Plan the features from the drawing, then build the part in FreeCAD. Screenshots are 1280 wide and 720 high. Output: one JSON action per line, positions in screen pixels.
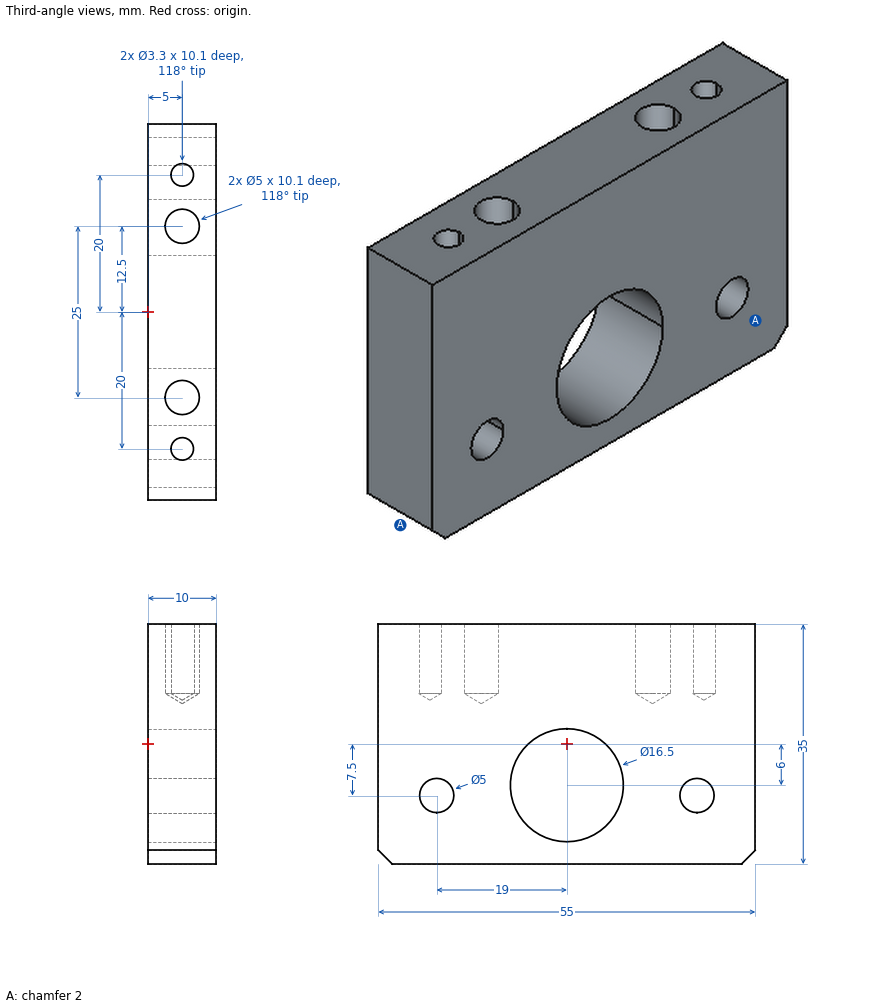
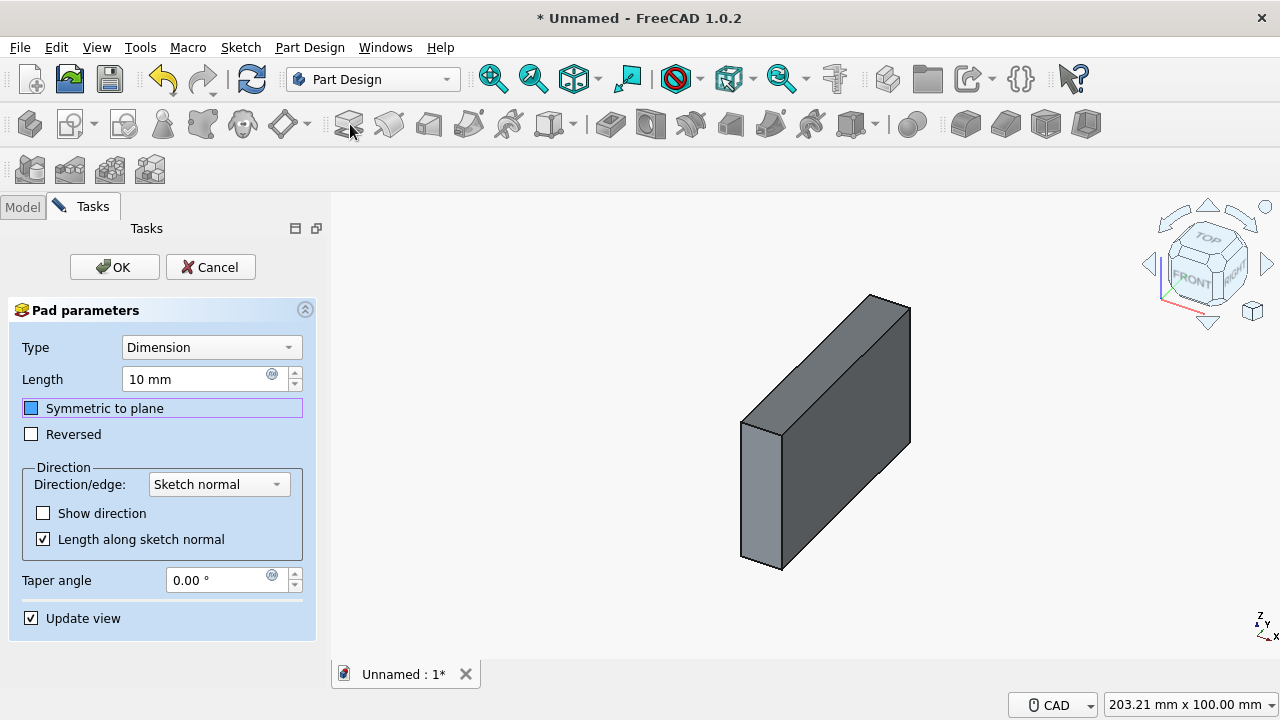
{"action": "left_click", "coordinate": [115, 267]}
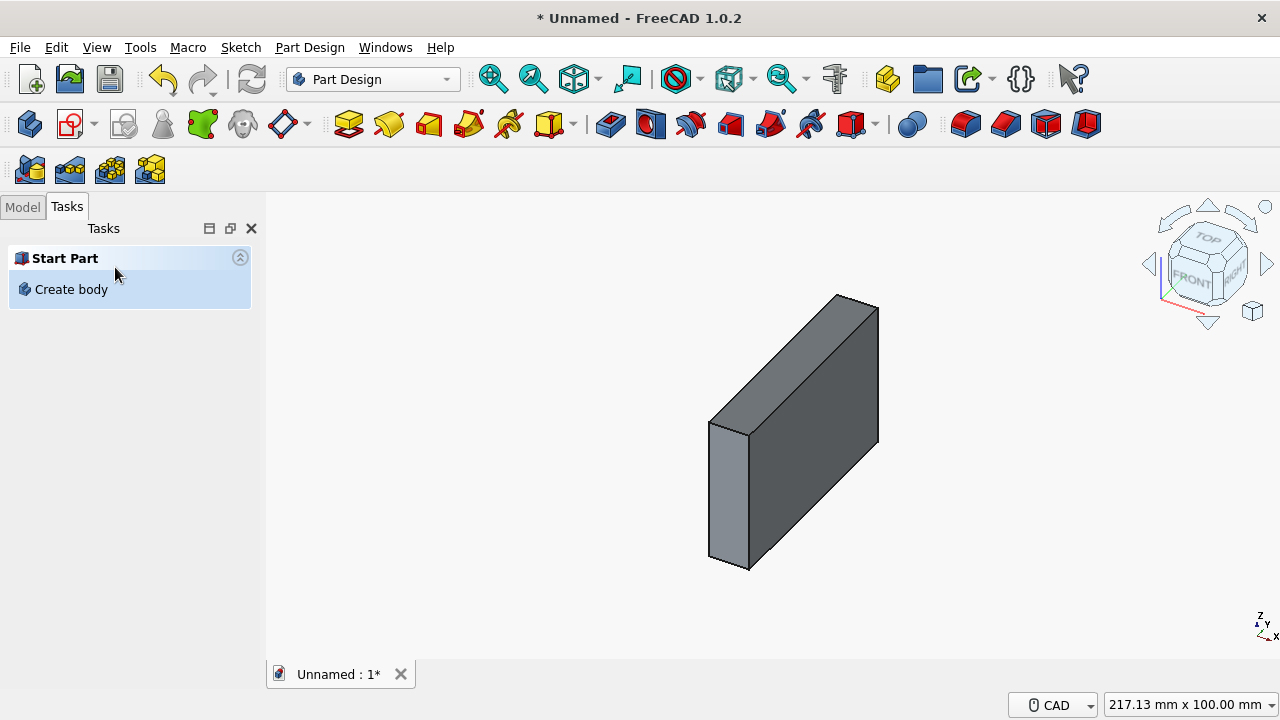
{"action": "left_click", "coordinate": [70, 124]}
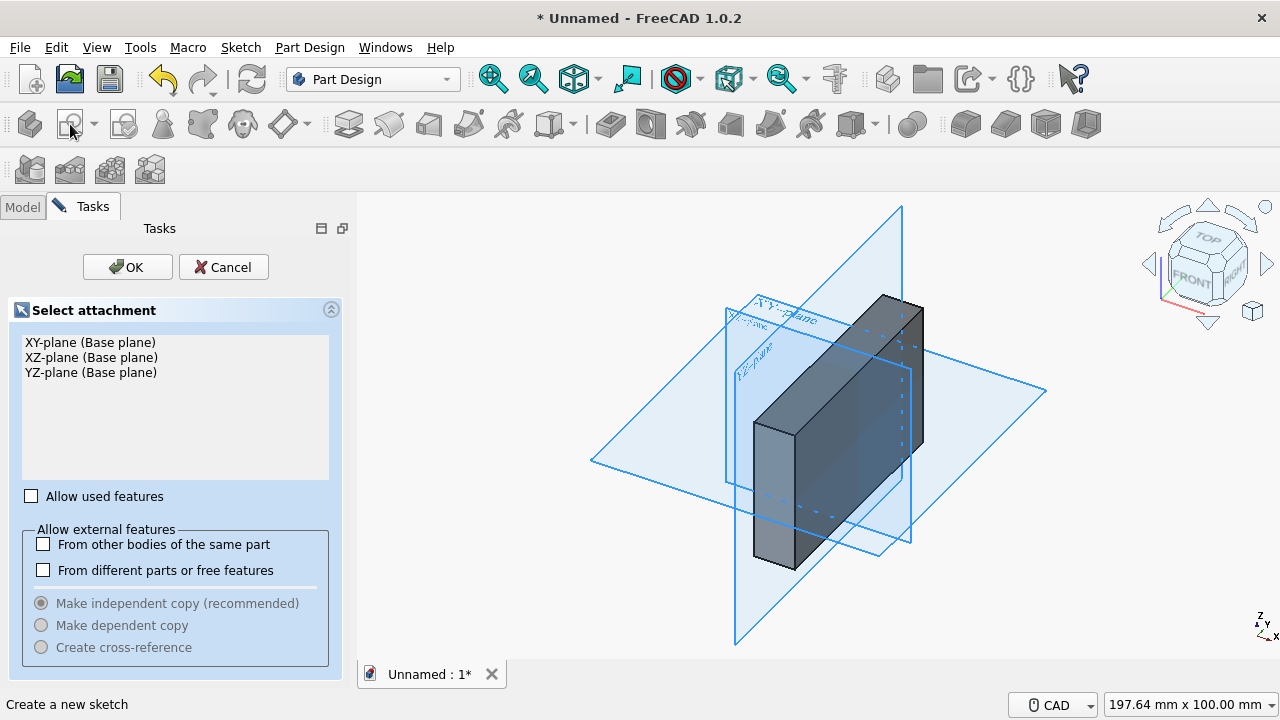
{"action": "left_click", "coordinate": [82, 372]}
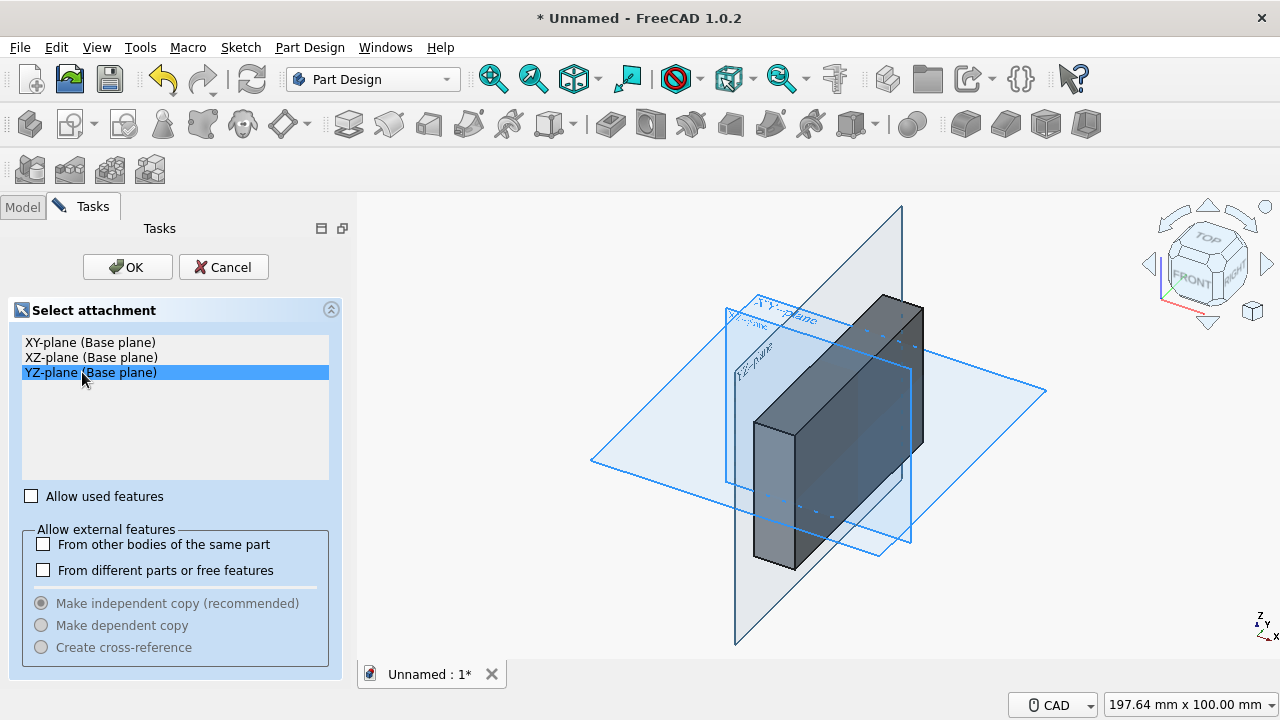
{"action": "left_click", "coordinate": [128, 267]}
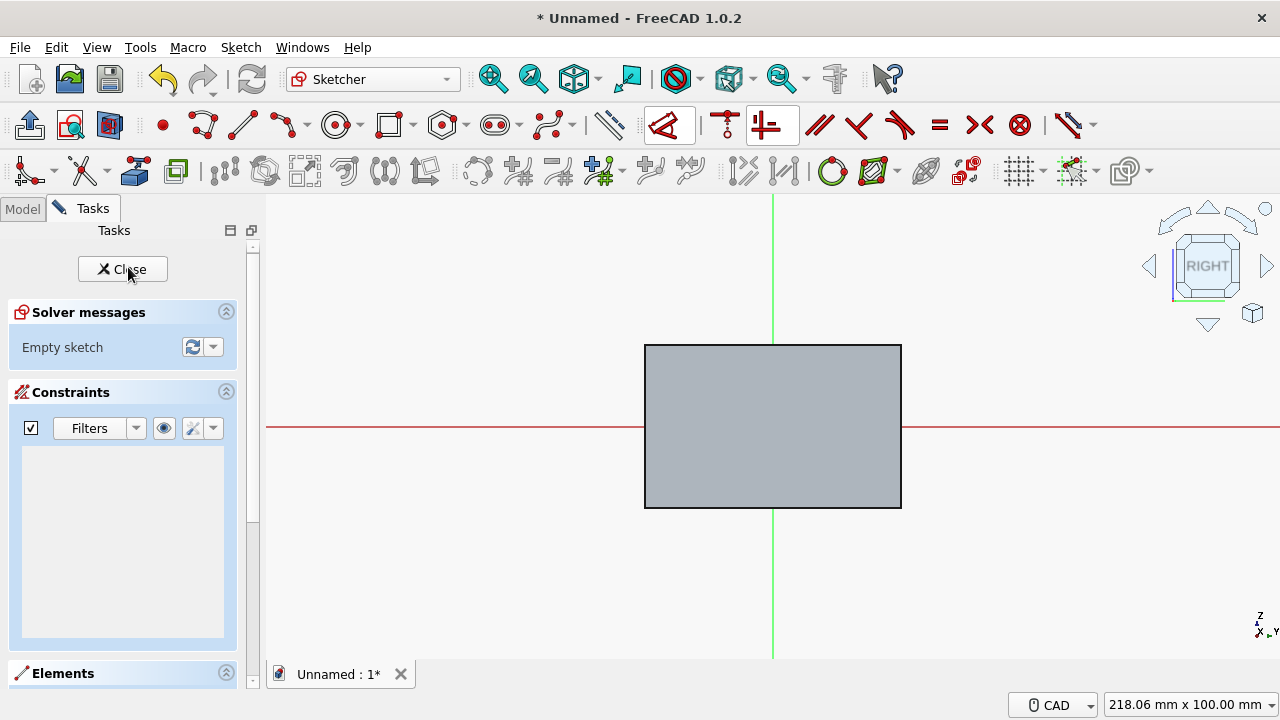
{"action": "left_click", "coordinate": [110, 126]}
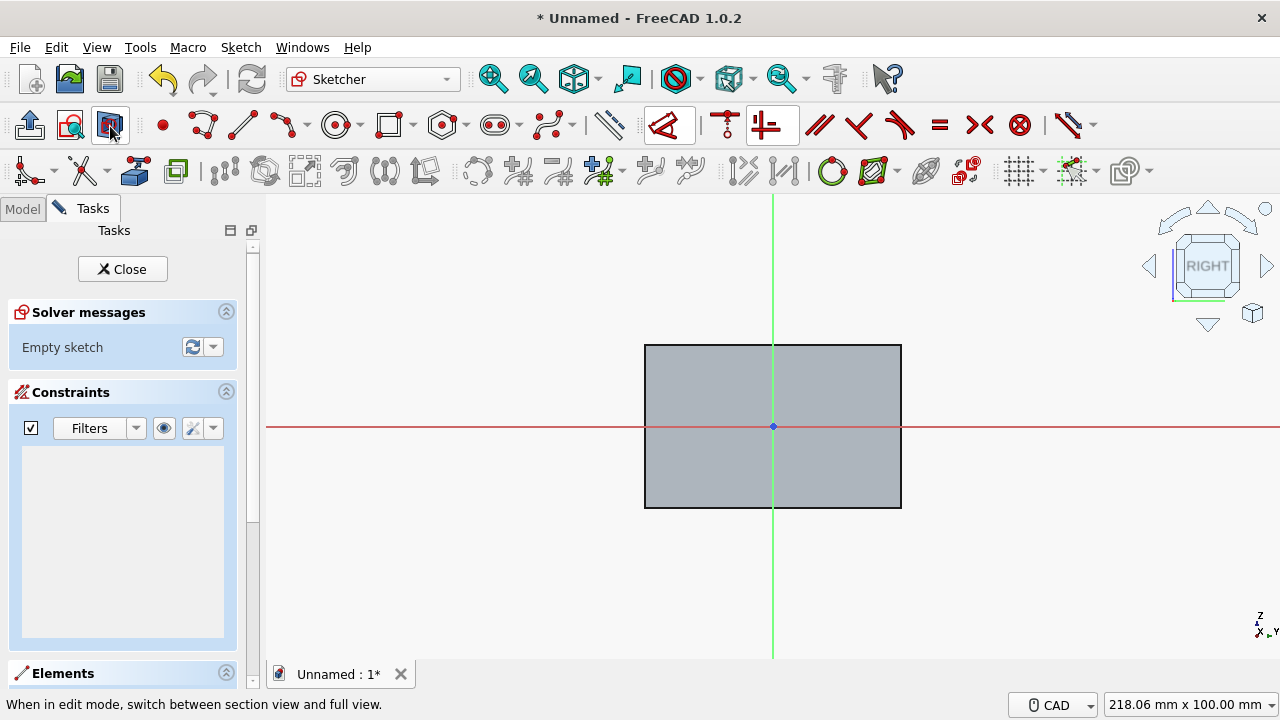
{"action": "scroll", "coordinate": [795, 464], "scroll_direction": "up", "scroll_amount": 7}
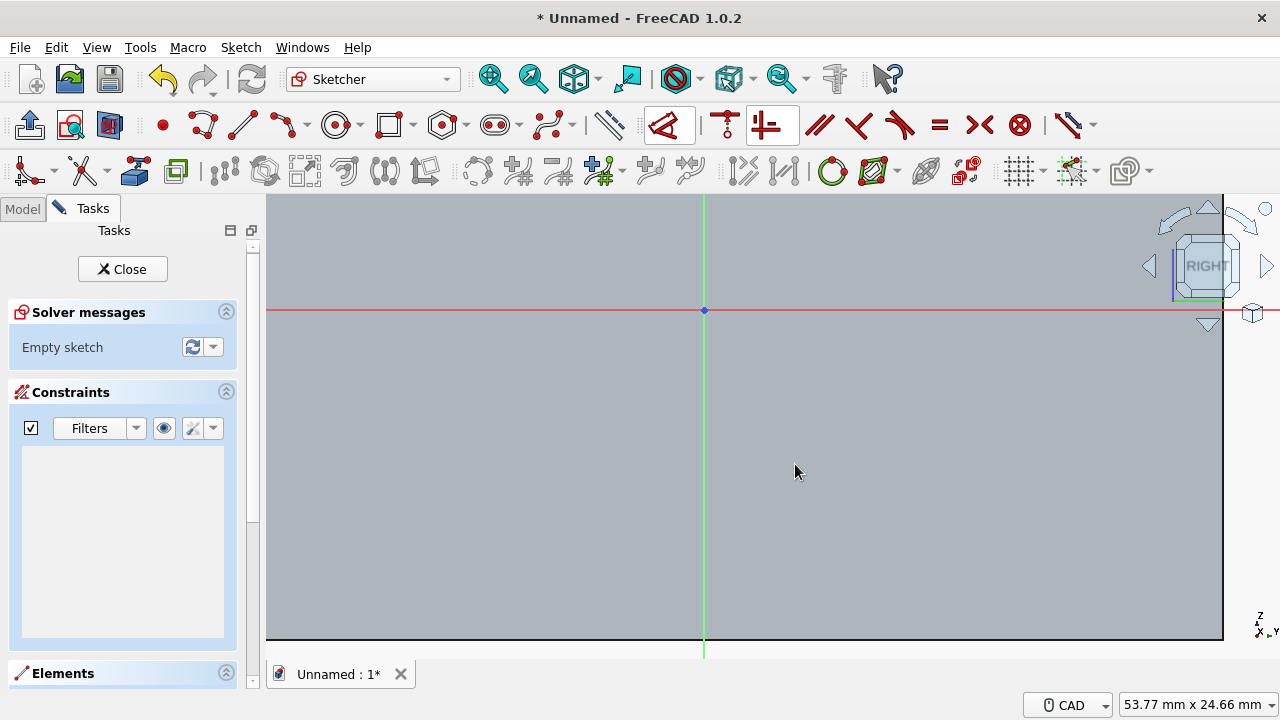
{"action": "left_click", "coordinate": [336, 126]}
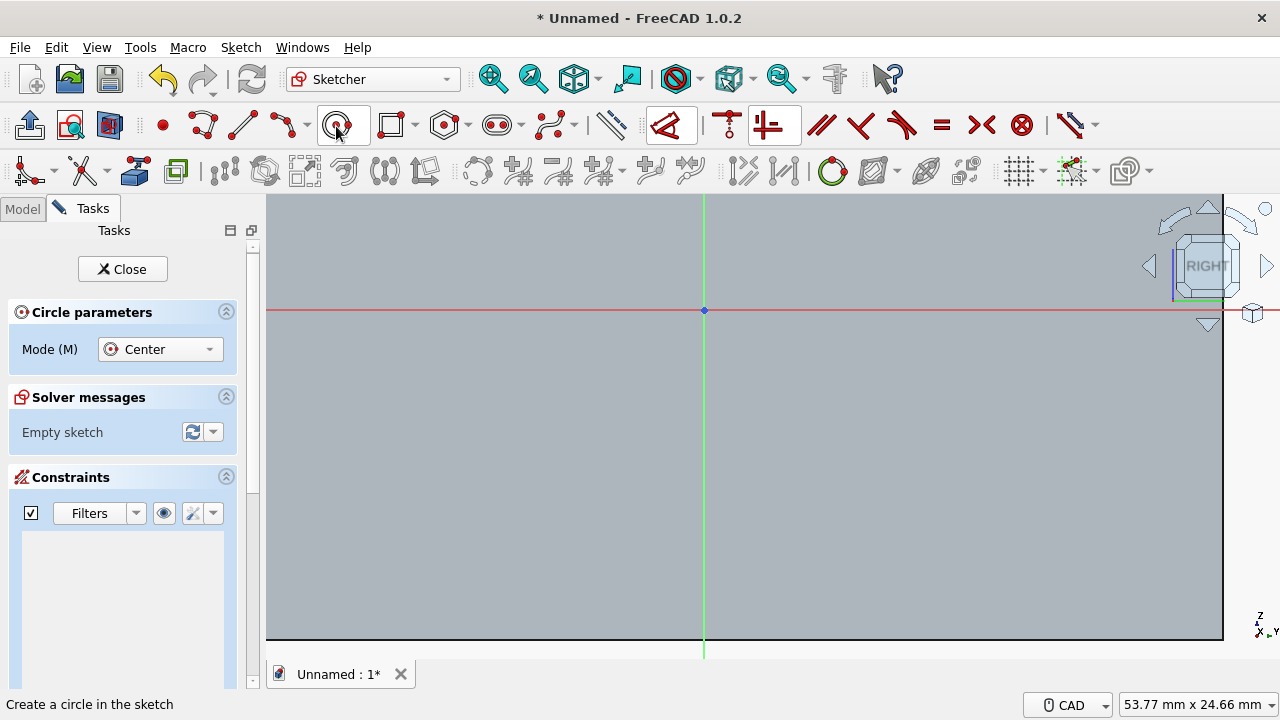
{"action": "left_click", "coordinate": [704, 423]}
{"action": "mouse_move", "coordinate": [814, 533]}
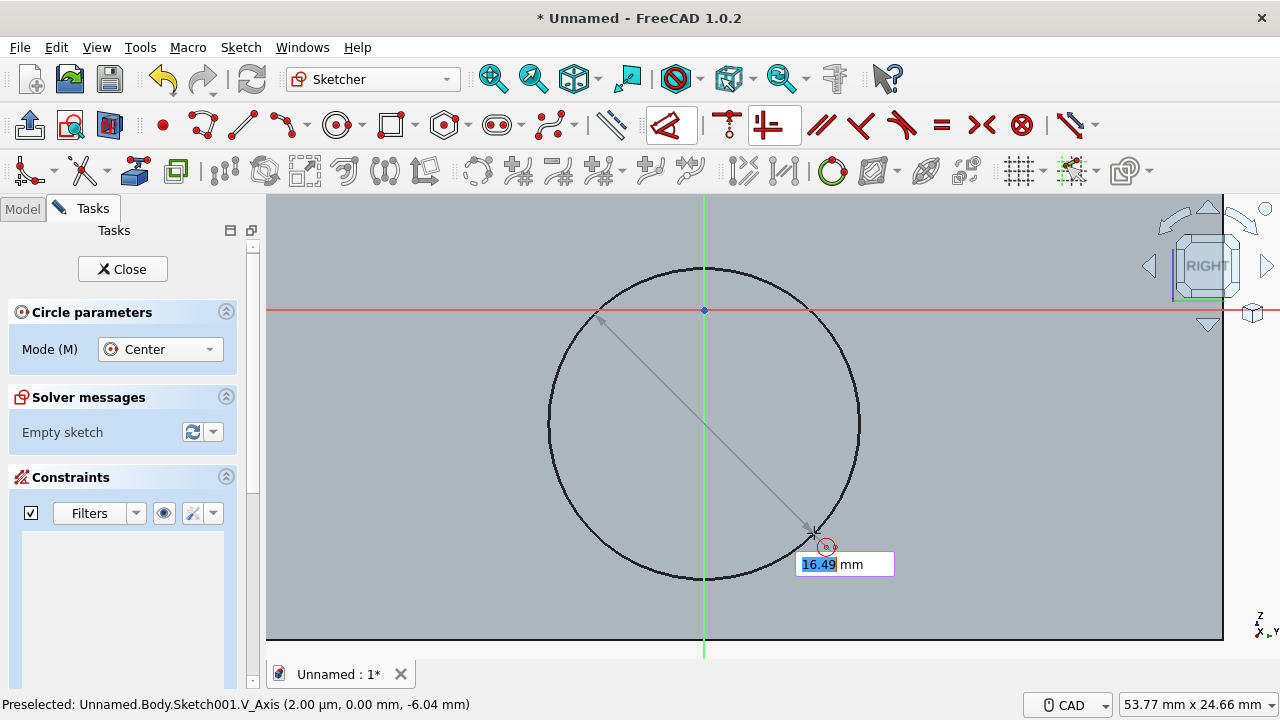
{"action": "type", "text": "16.5"}
{"action": "key", "text": "Return"}
{"action": "key", "text": "Escape"}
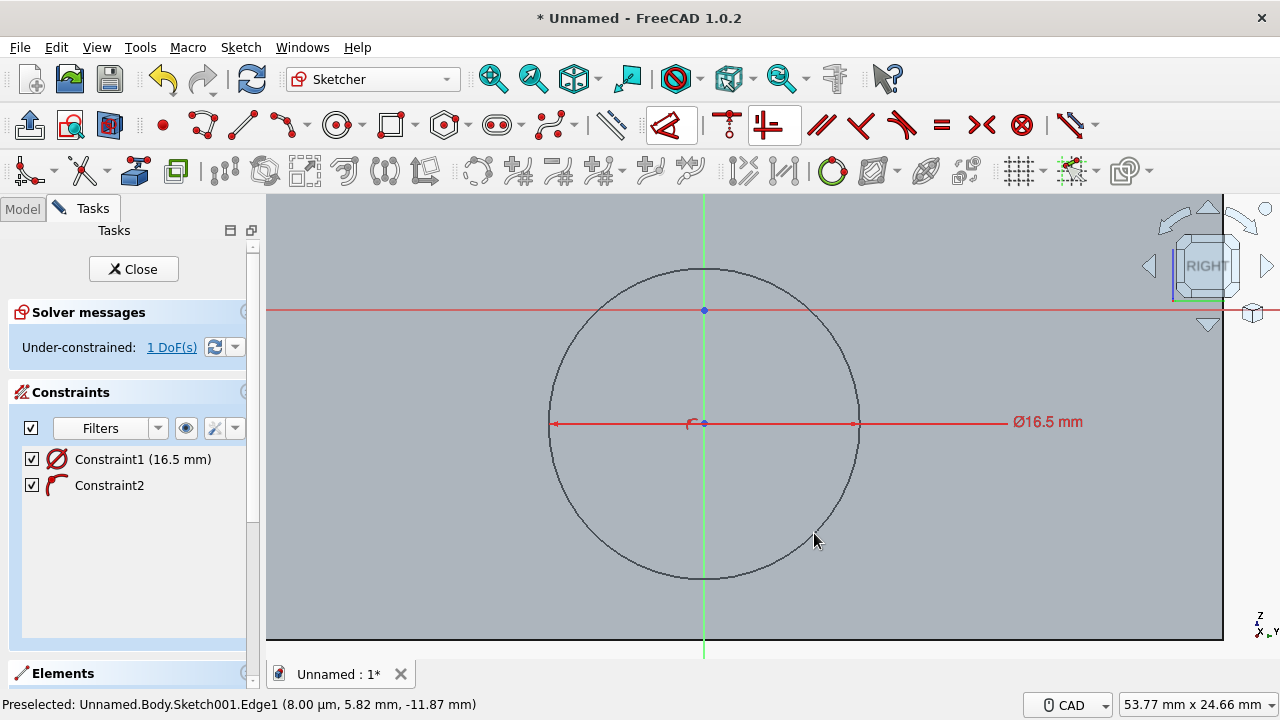
{"action": "left_click", "coordinate": [666, 126]}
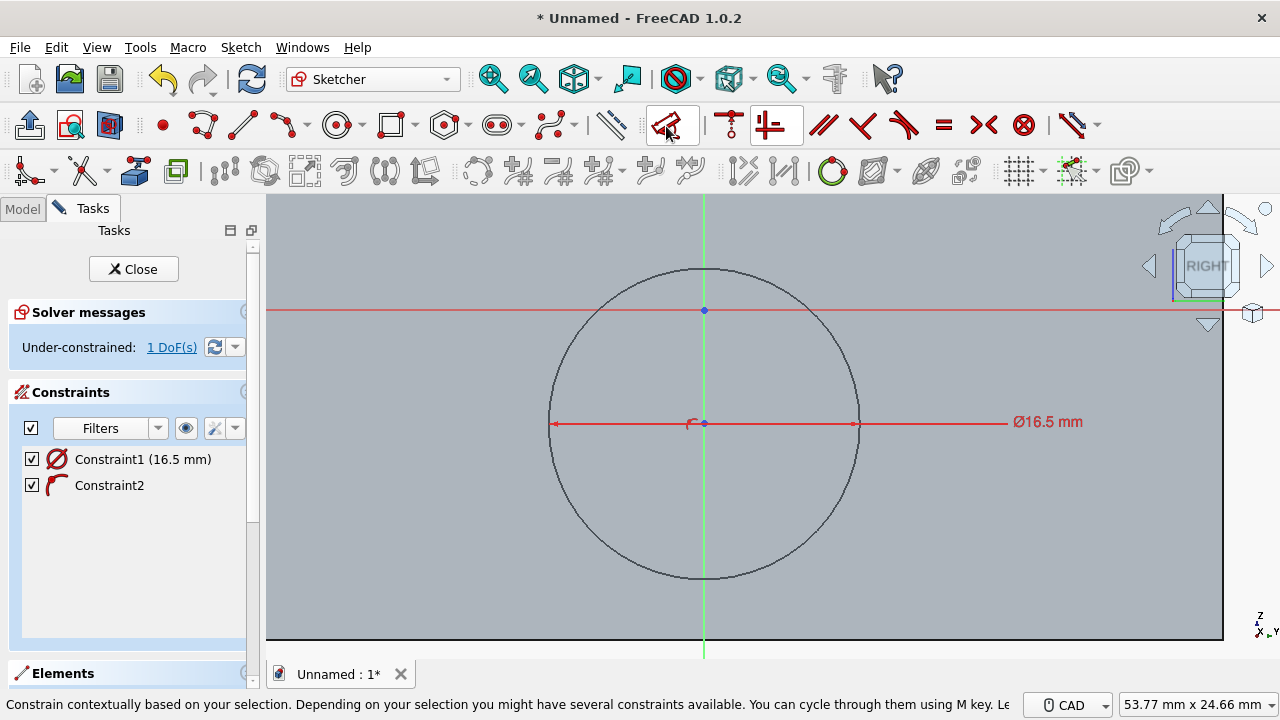
{"action": "left_click", "coordinate": [704, 424]}
{"action": "left_click", "coordinate": [738, 367]}